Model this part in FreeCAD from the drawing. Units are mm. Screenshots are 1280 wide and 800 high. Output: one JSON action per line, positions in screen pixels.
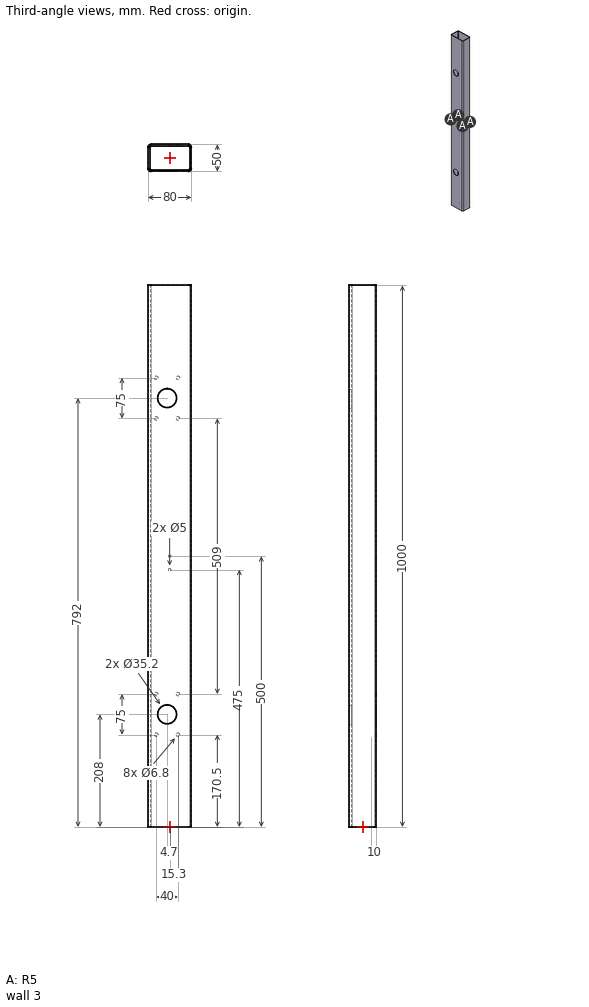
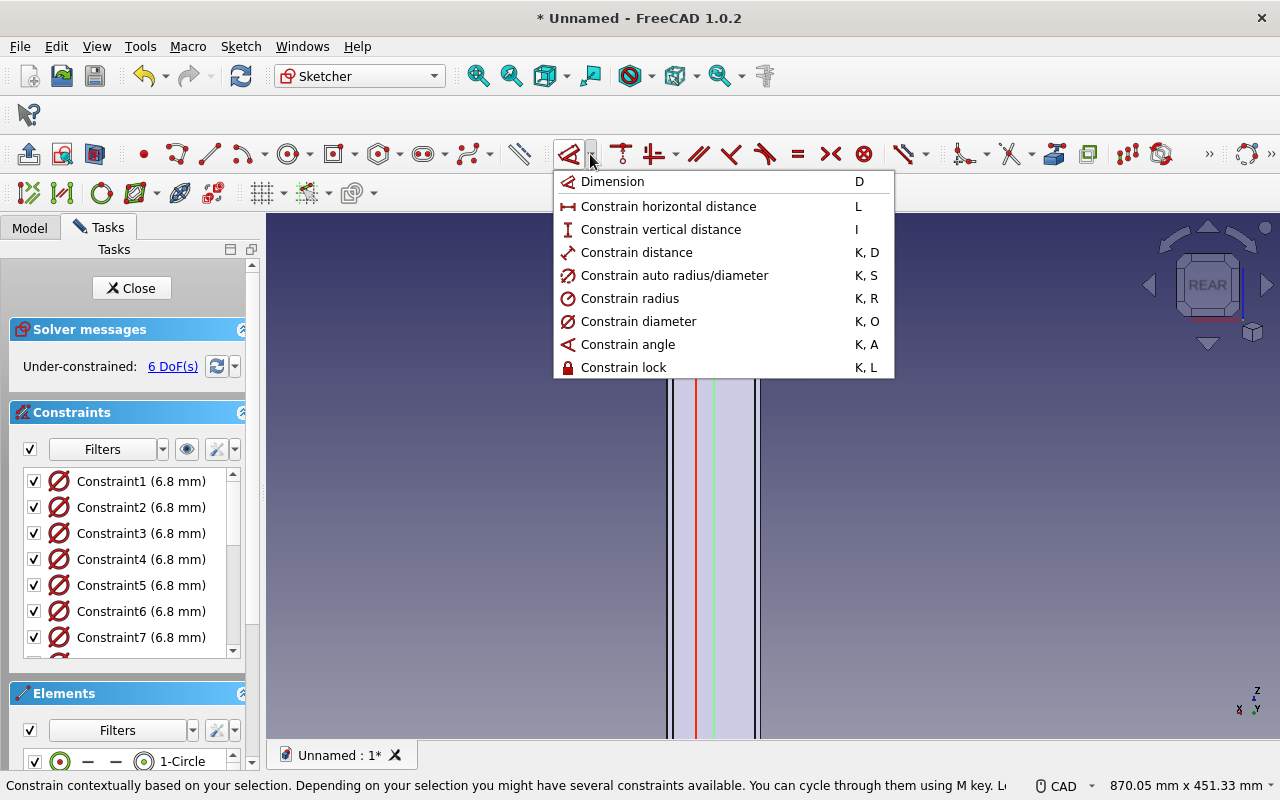
{"action": "left_click", "coordinate": [724, 230]}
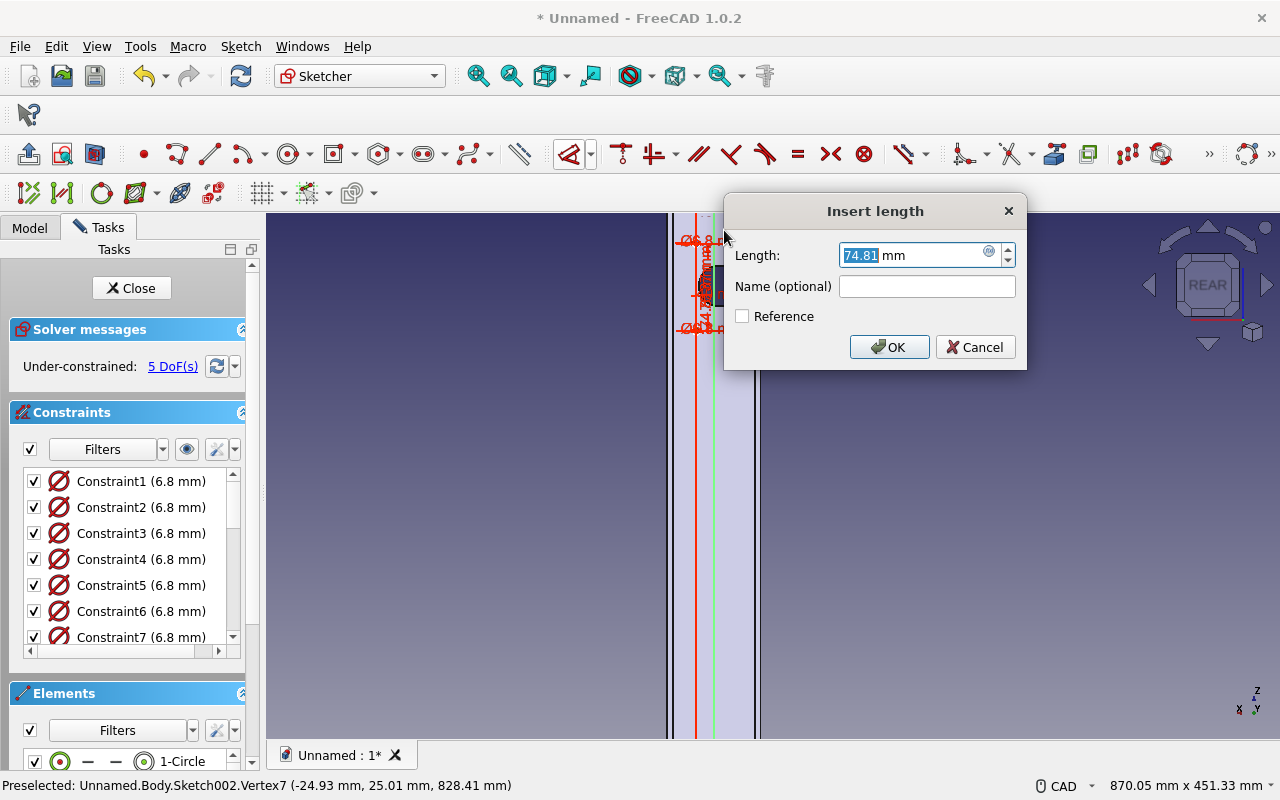
{"action": "type", "text": "75"}
{"action": "key", "text": "Return"}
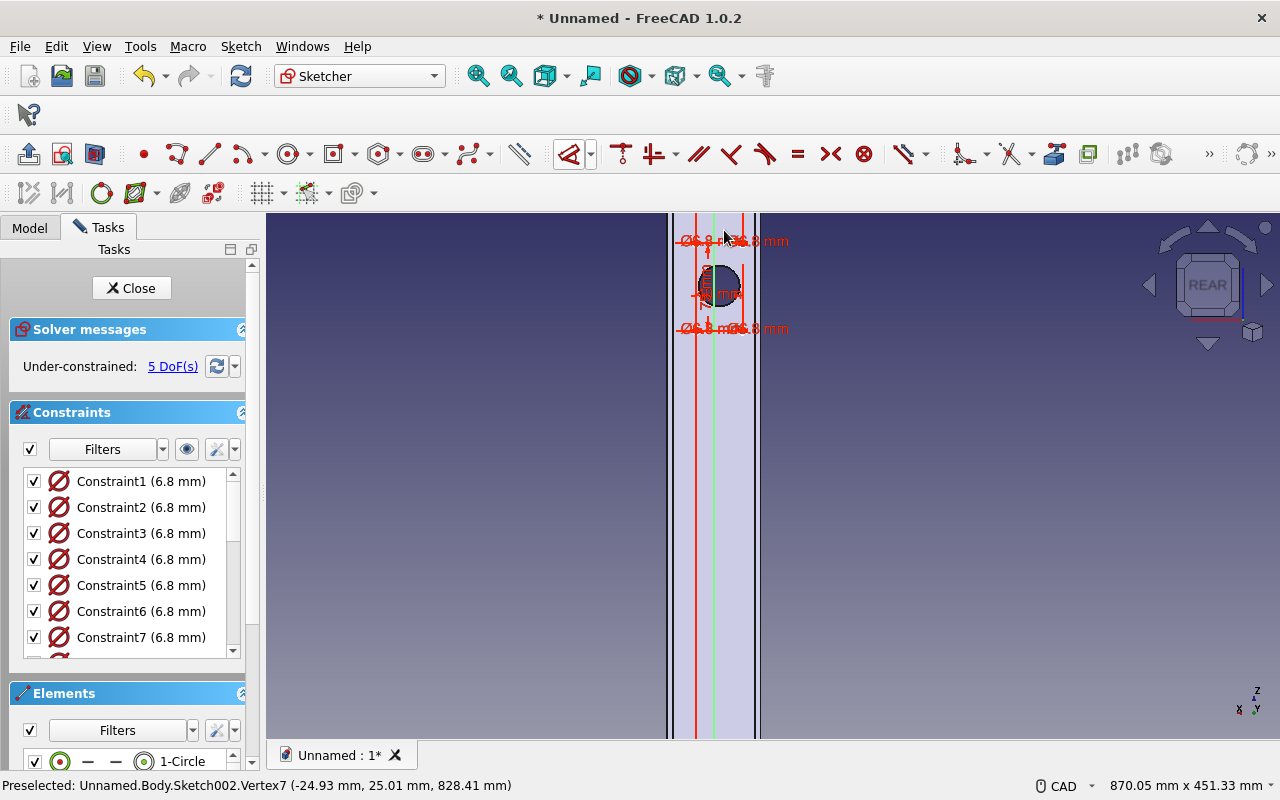
{"action": "left_click", "coordinate": [743, 243]}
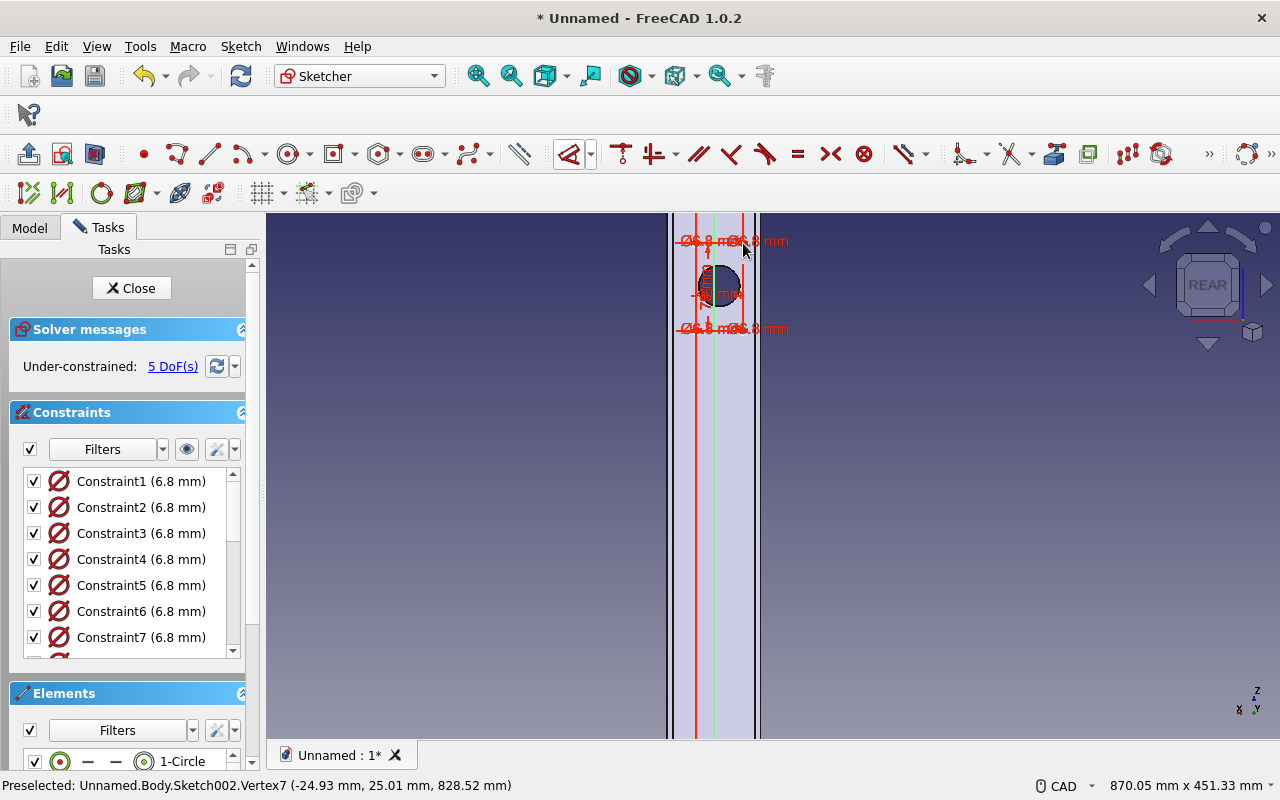
{"action": "left_click", "coordinate": [696, 243]}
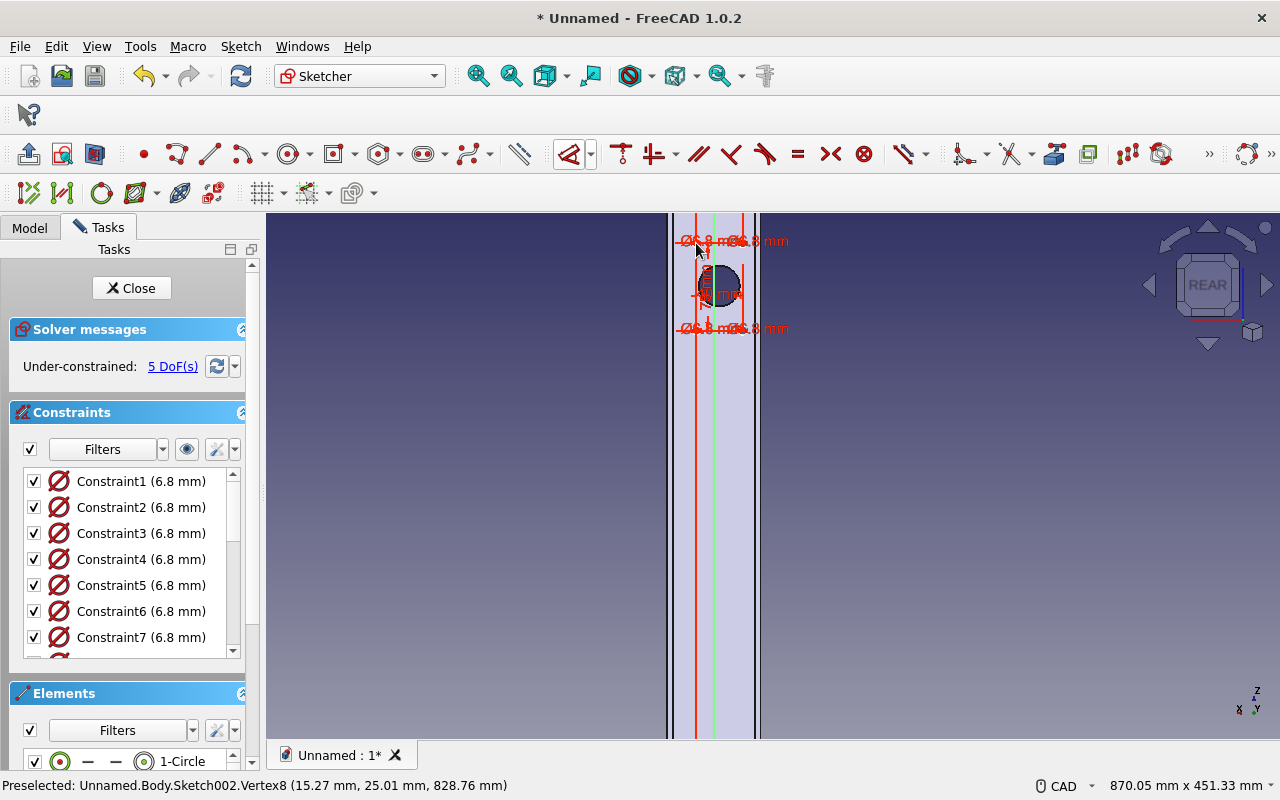
{"action": "key", "text": "l"}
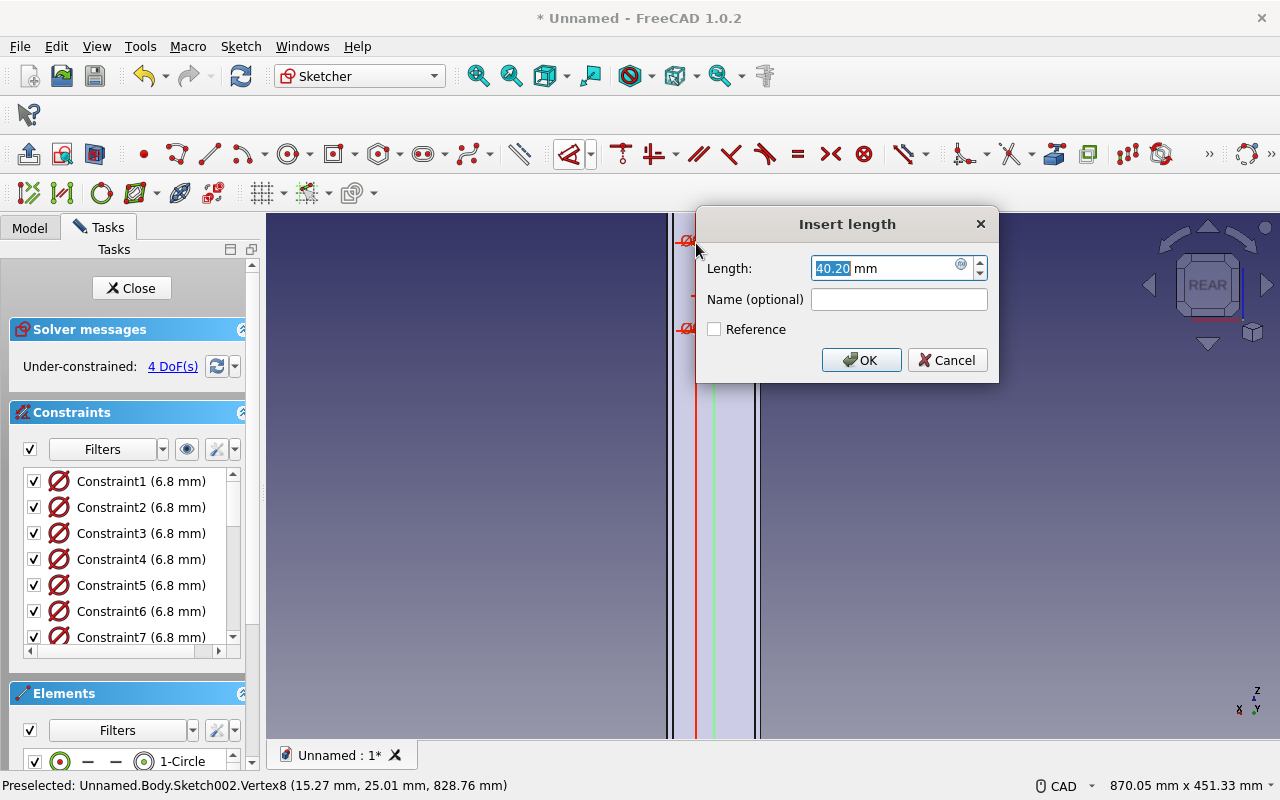
{"action": "type", "text": "40"}
{"action": "key", "text": "Return"}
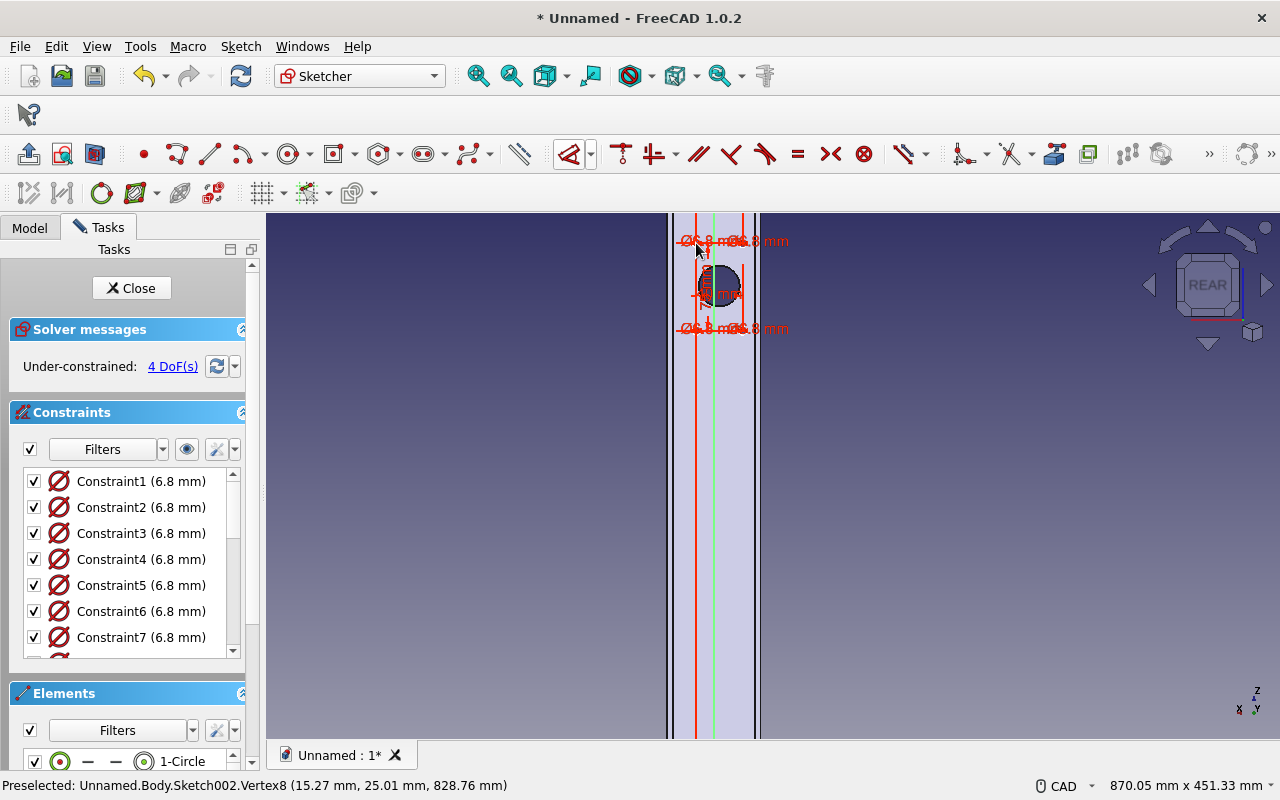
{"action": "left_click", "coordinate": [696, 331]}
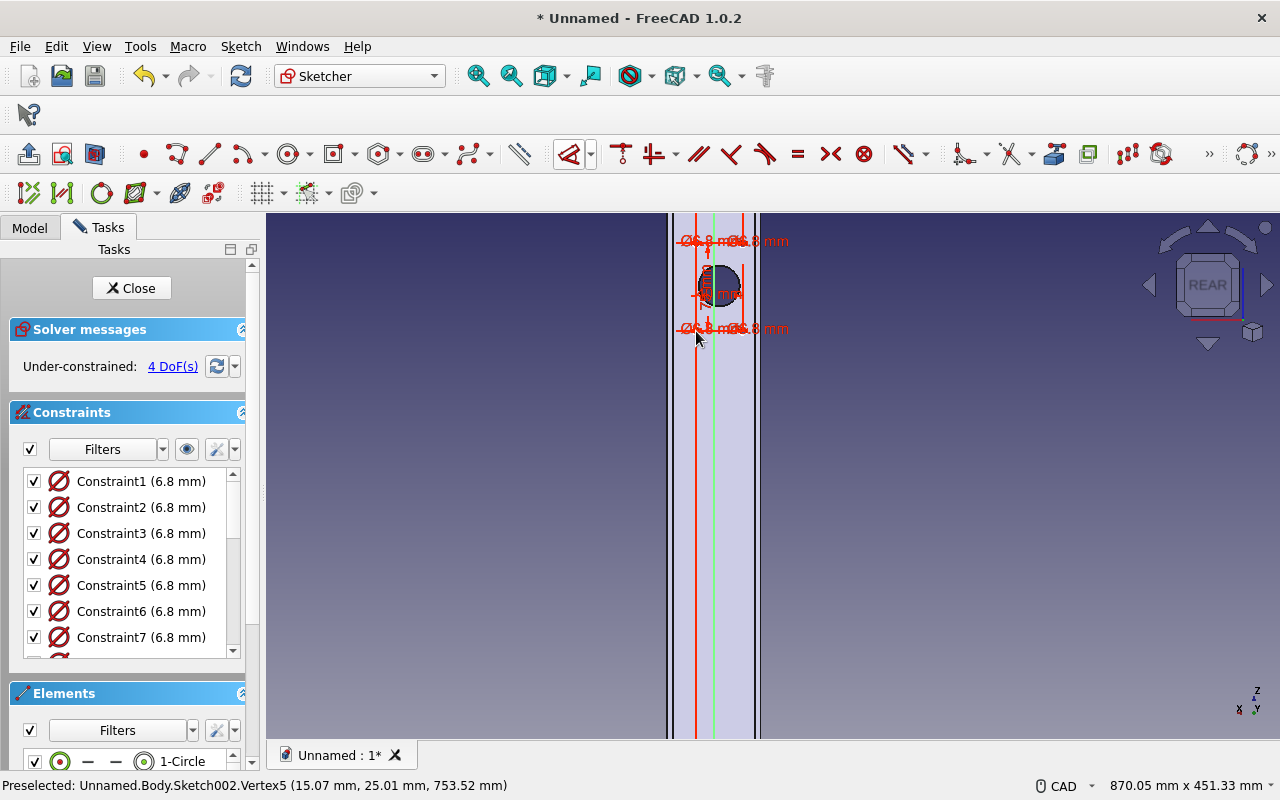
{"action": "left_click", "coordinate": [696, 243]}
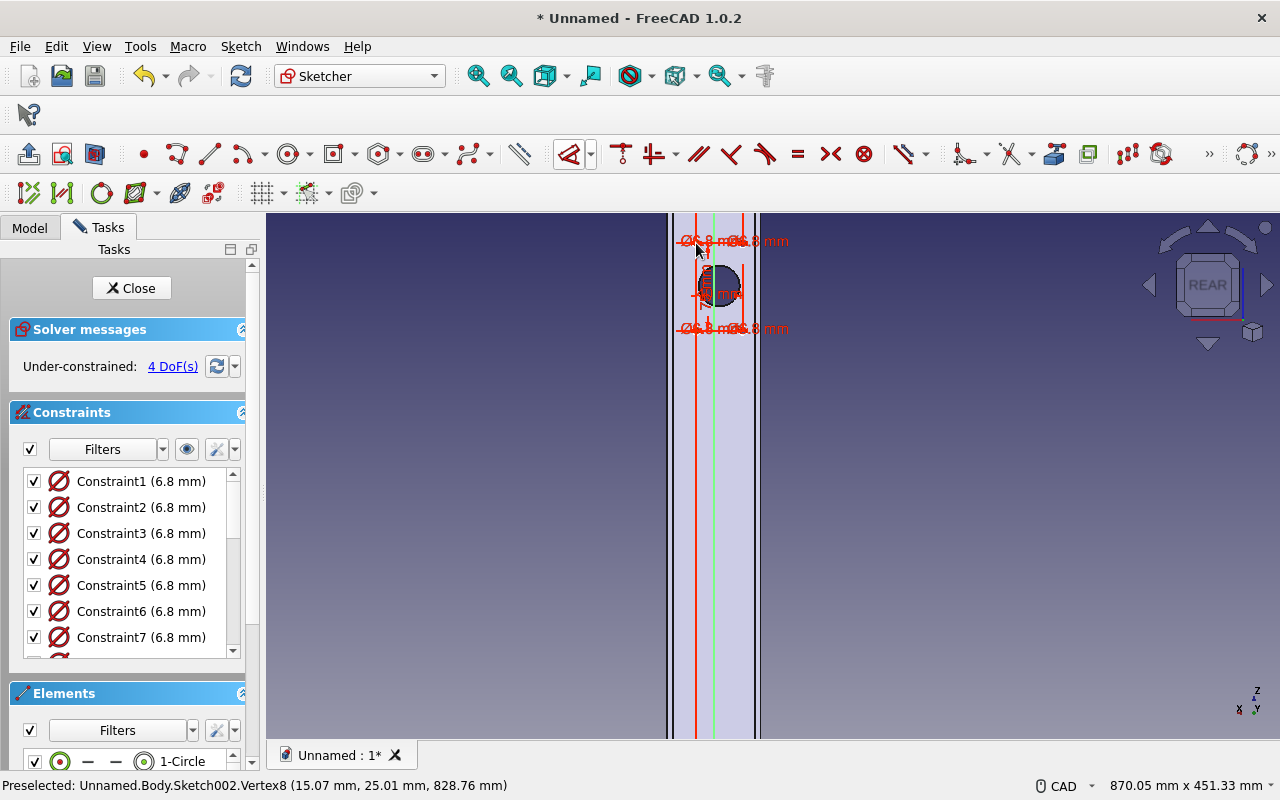
{"action": "left_click", "coordinate": [590, 154]}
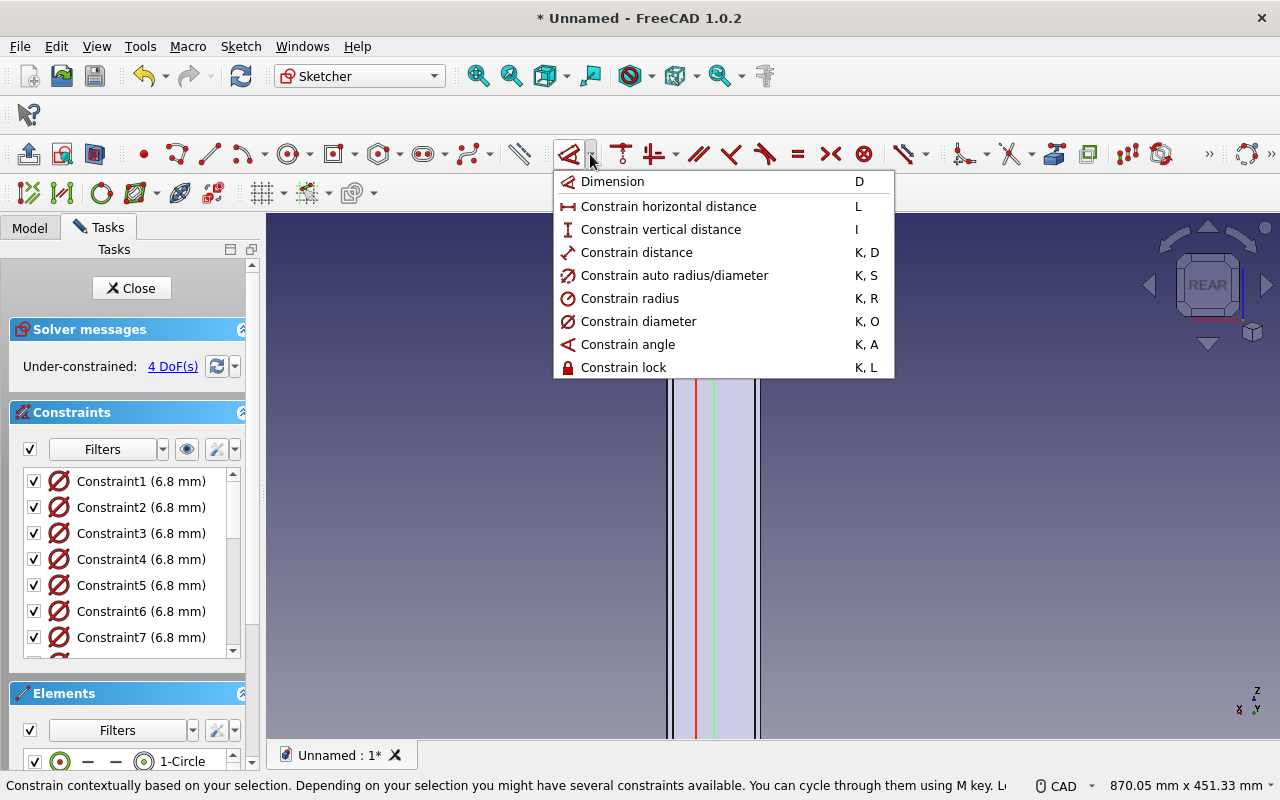
{"action": "left_click", "coordinate": [724, 230]}